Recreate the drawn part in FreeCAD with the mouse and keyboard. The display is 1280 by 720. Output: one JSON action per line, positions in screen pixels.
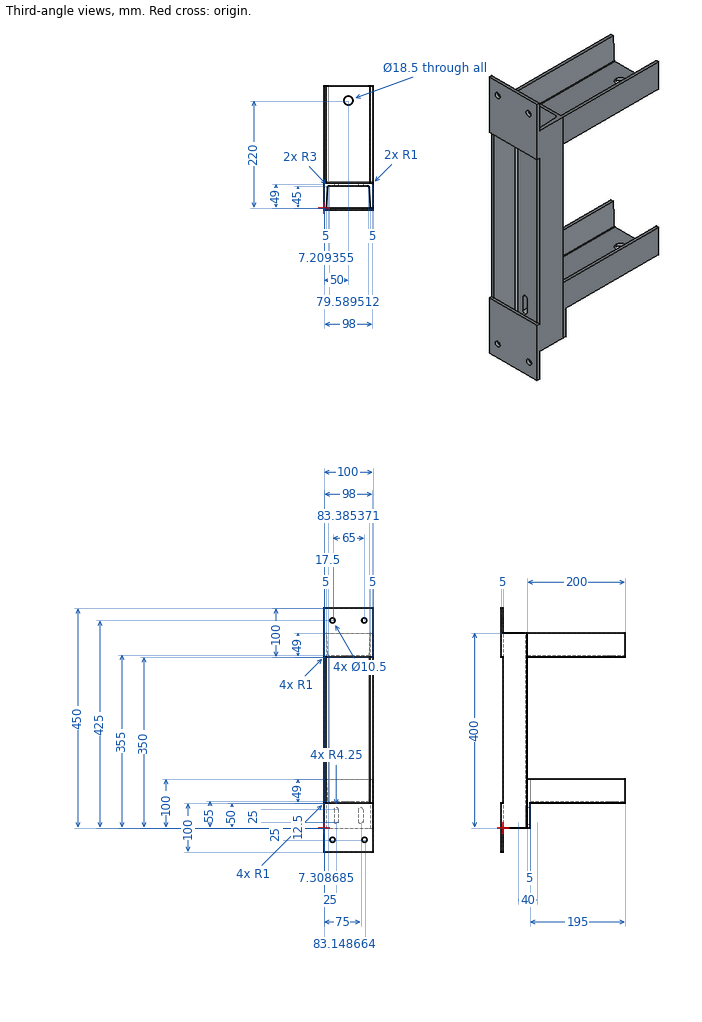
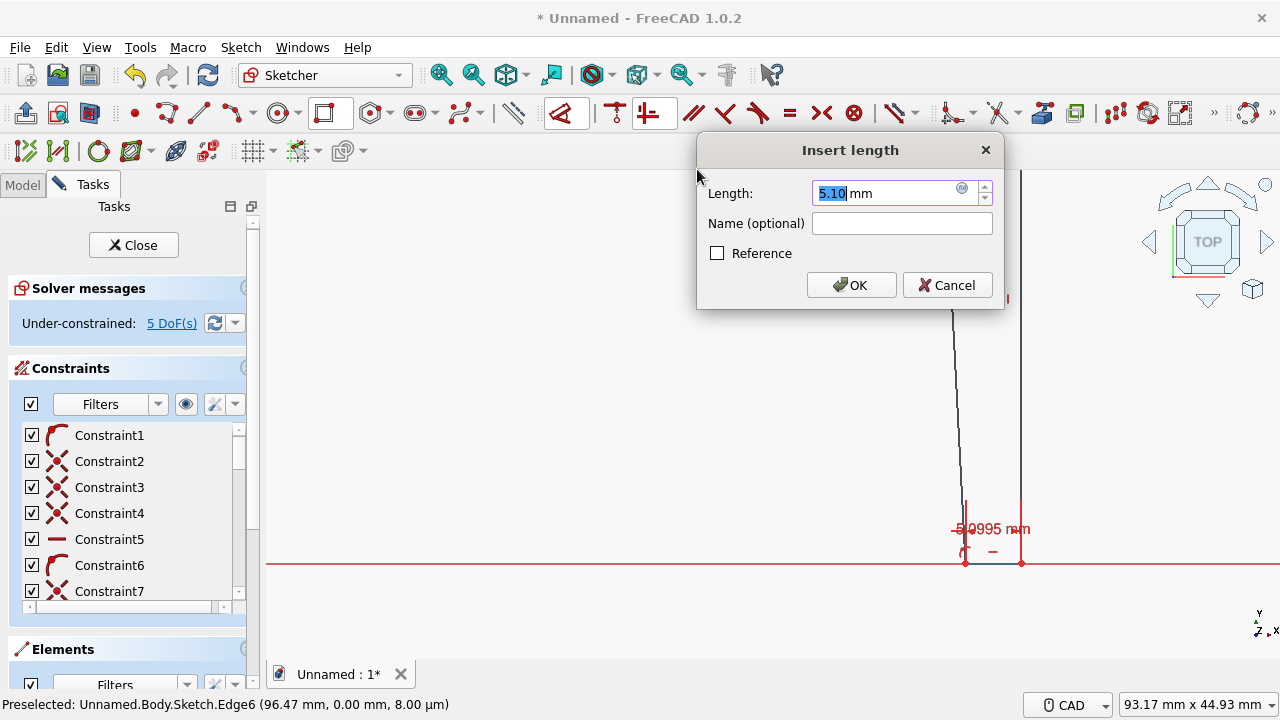
{"action": "type", "text": "5"}
{"action": "key", "text": "Return"}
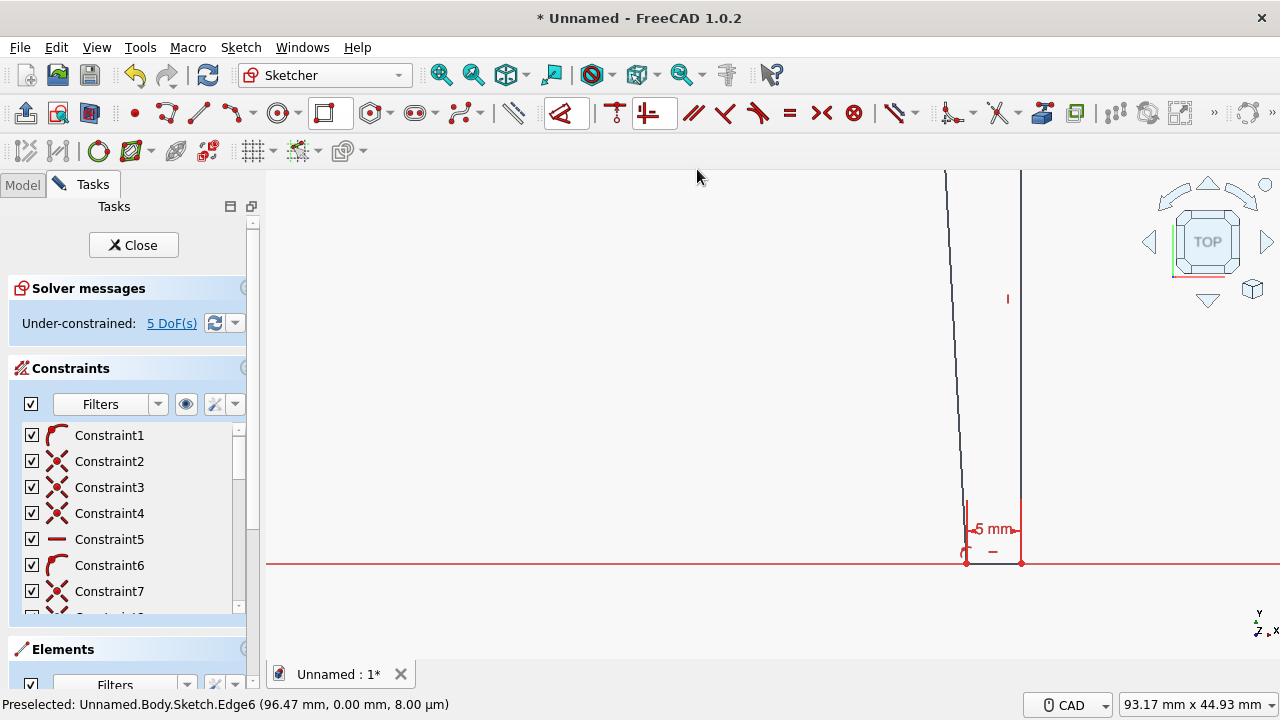
{"action": "scroll", "coordinate": [982, 564], "scroll_direction": "down", "scroll_amount": 3}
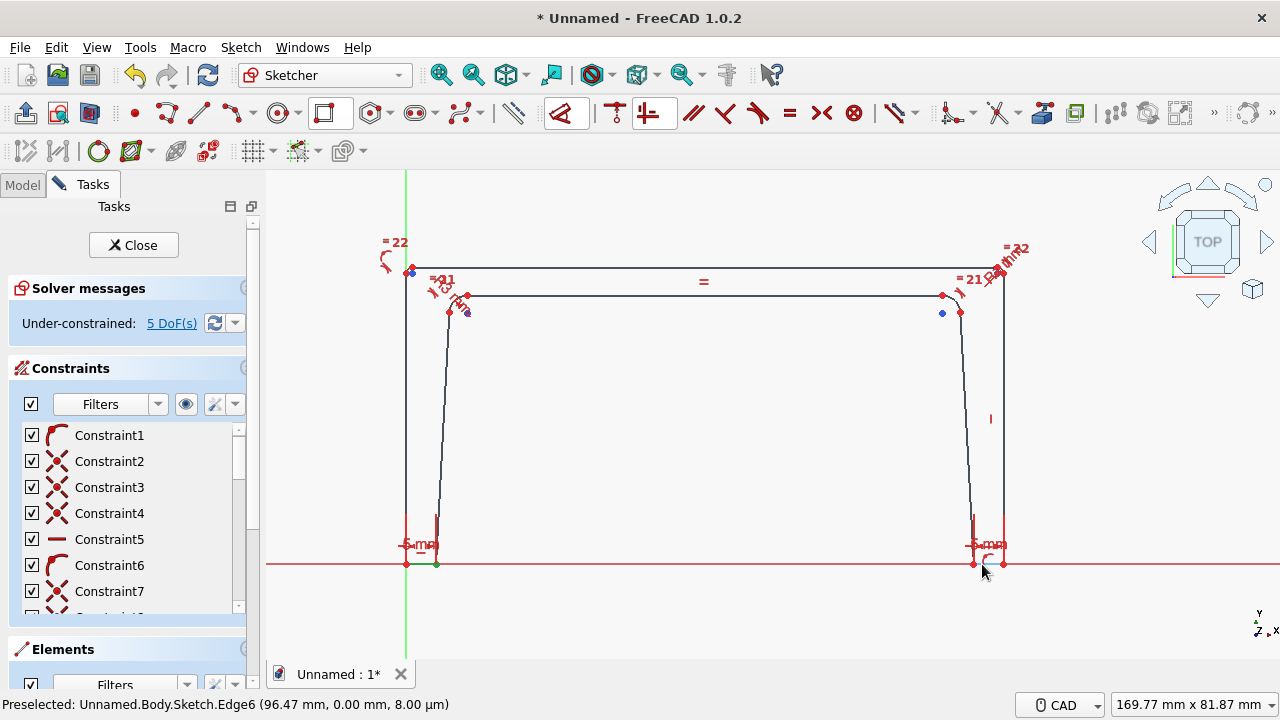
{"action": "left_click", "coordinate": [406, 361]}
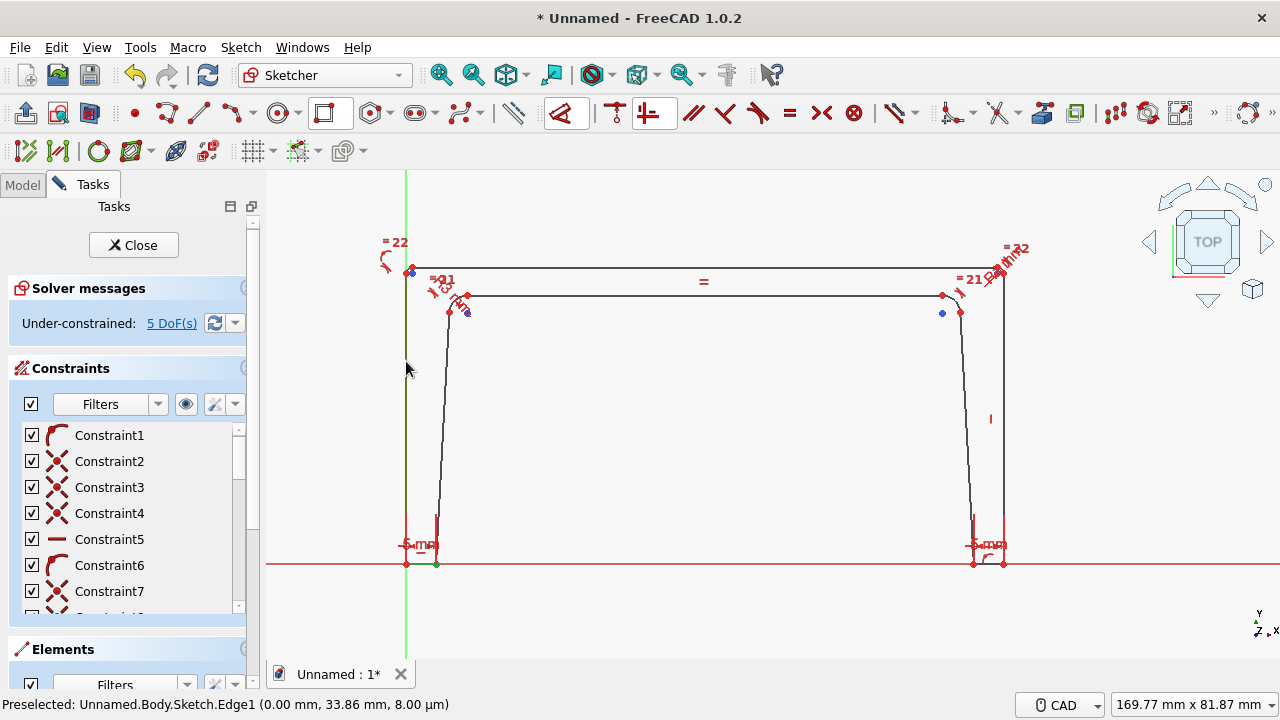
{"action": "left_click", "coordinate": [584, 114]}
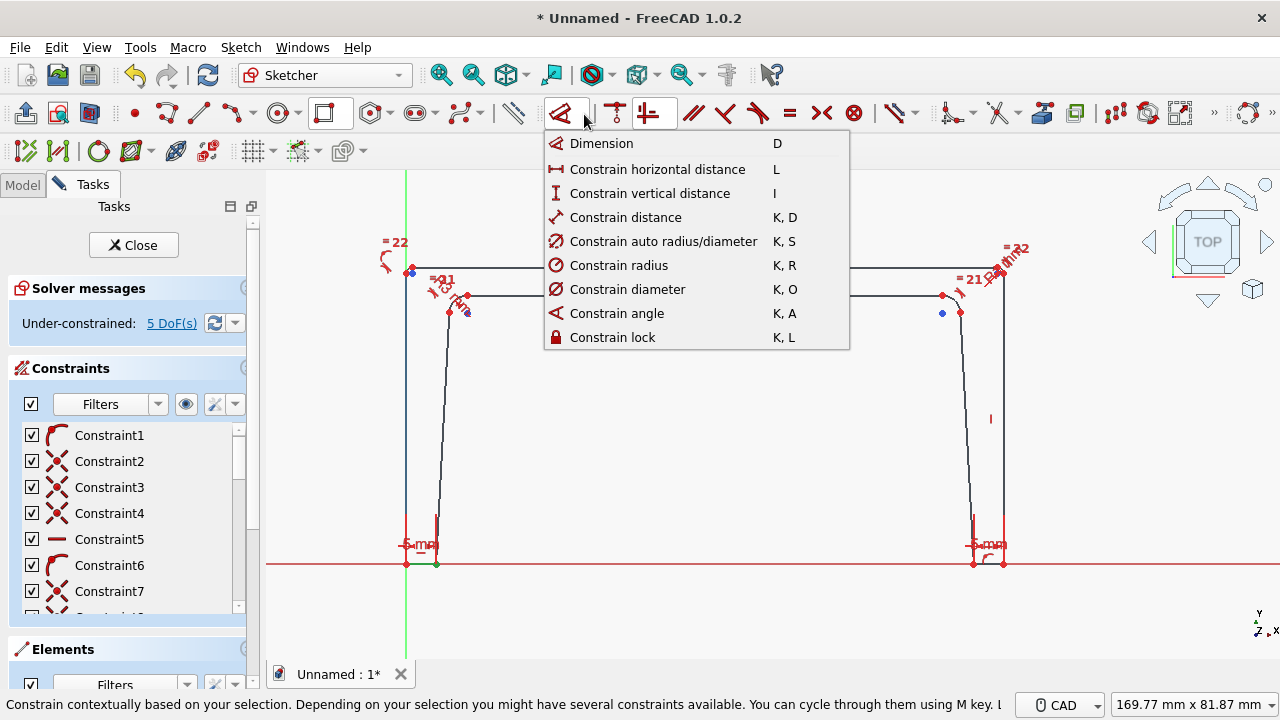
{"action": "left_click", "coordinate": [697, 193]}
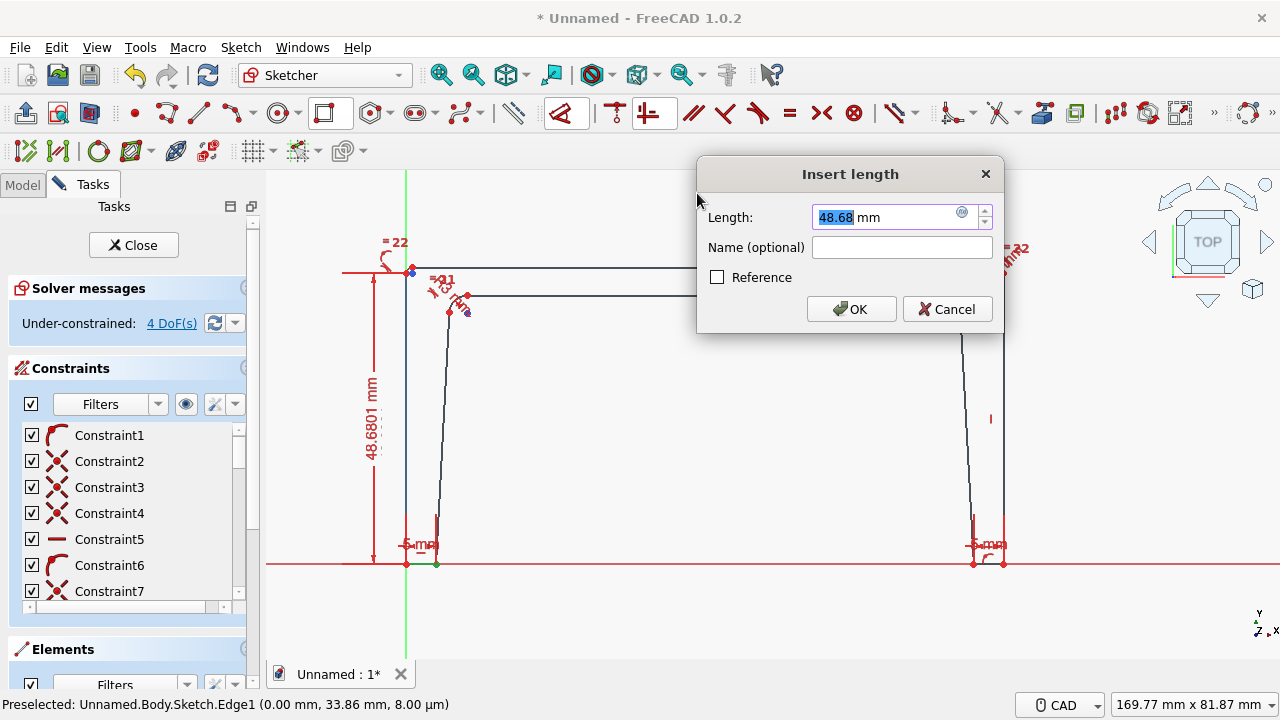
{"action": "type", "text": "49"}
{"action": "key", "text": "Return"}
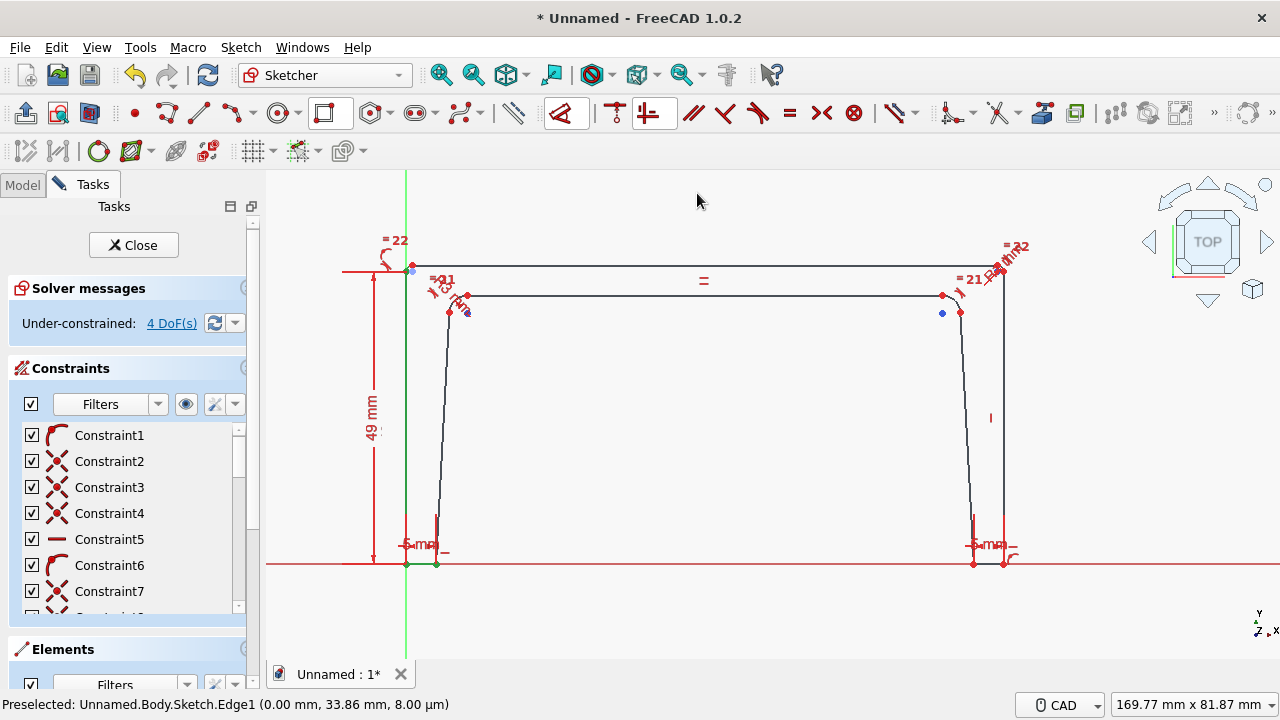
{"action": "left_click", "coordinate": [822, 266]}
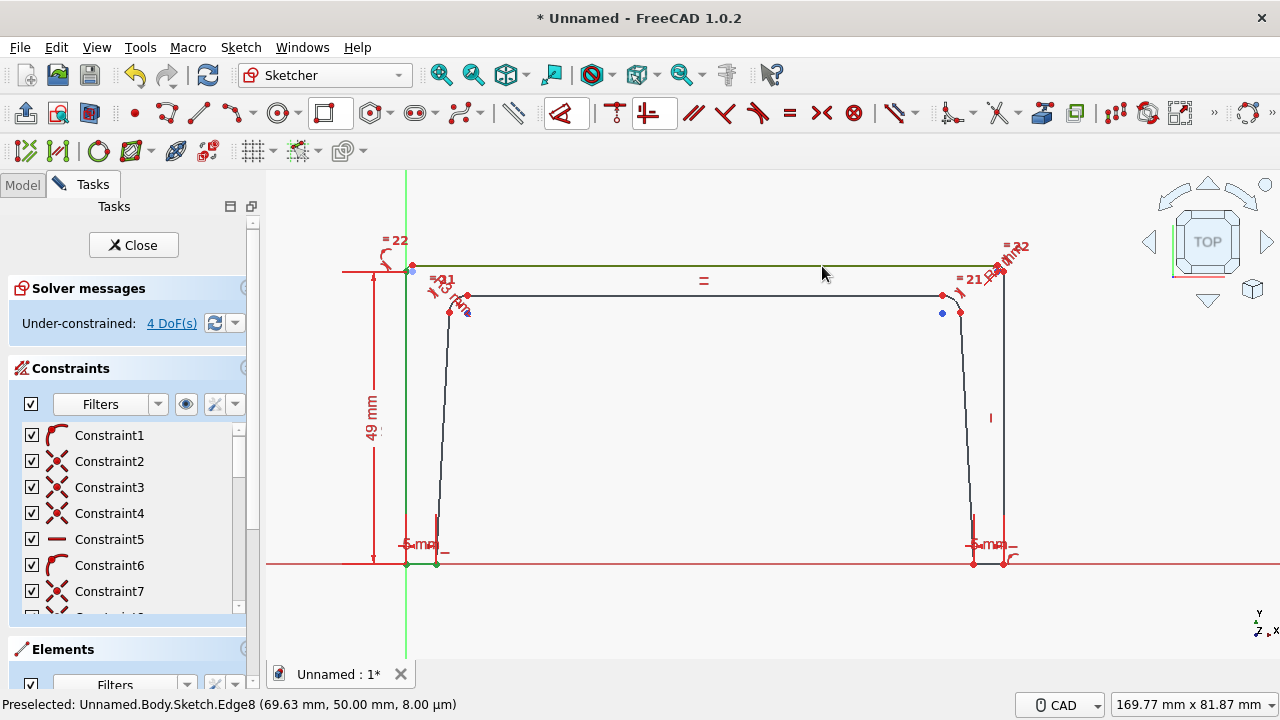
{"action": "key", "text": "l"}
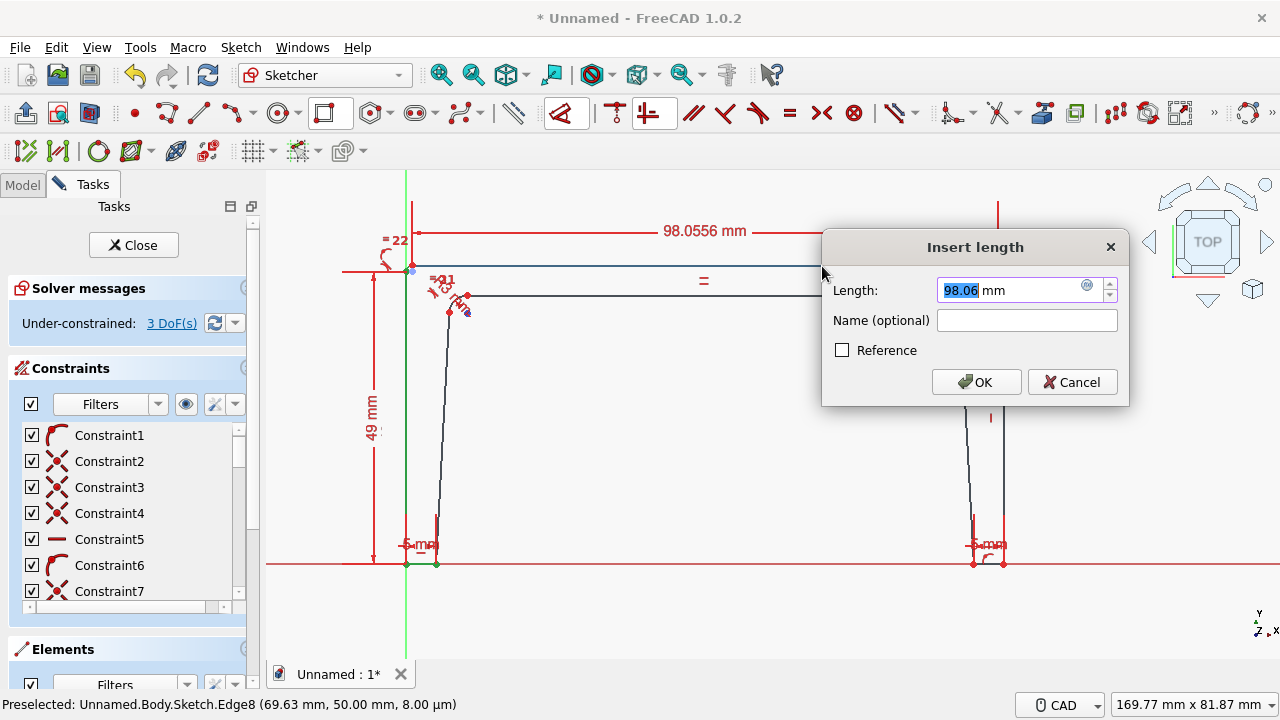
{"action": "type", "text": "98"}
{"action": "key", "text": "Return"}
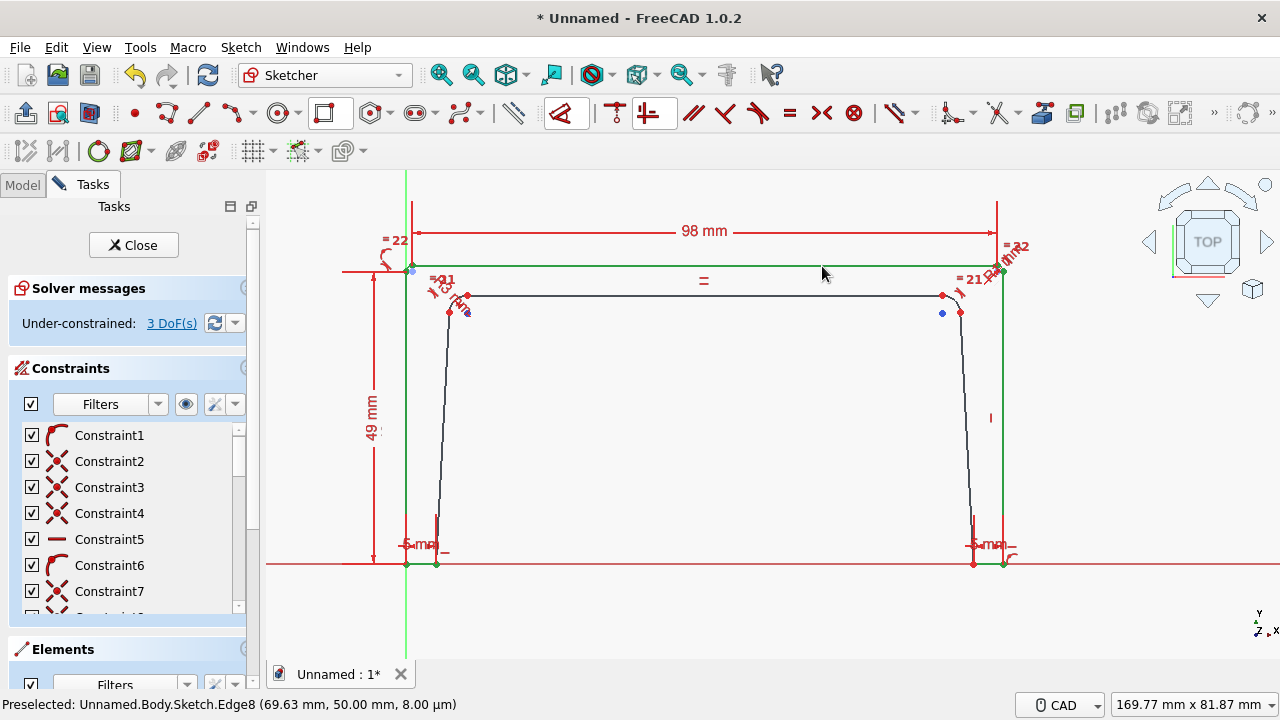
{"action": "left_click", "coordinate": [467, 296]}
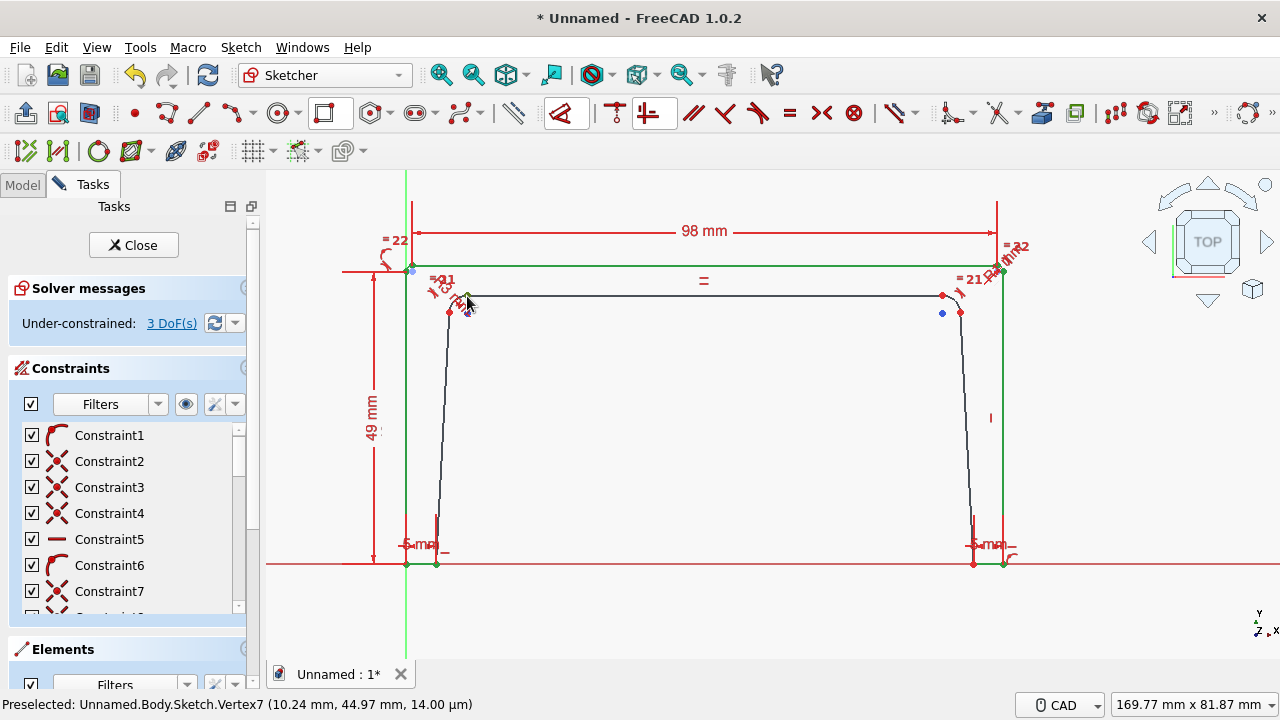
{"action": "key", "text": "i"}